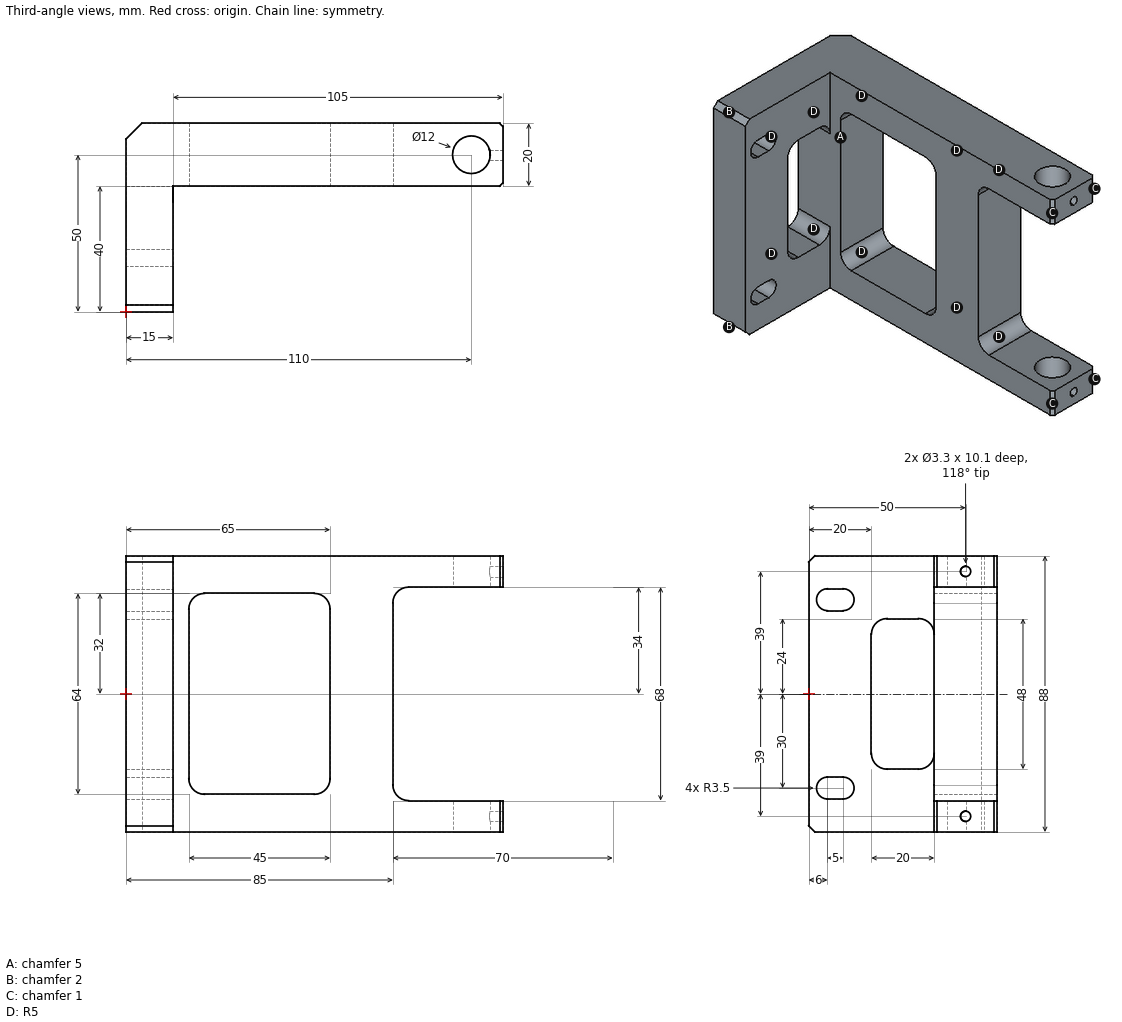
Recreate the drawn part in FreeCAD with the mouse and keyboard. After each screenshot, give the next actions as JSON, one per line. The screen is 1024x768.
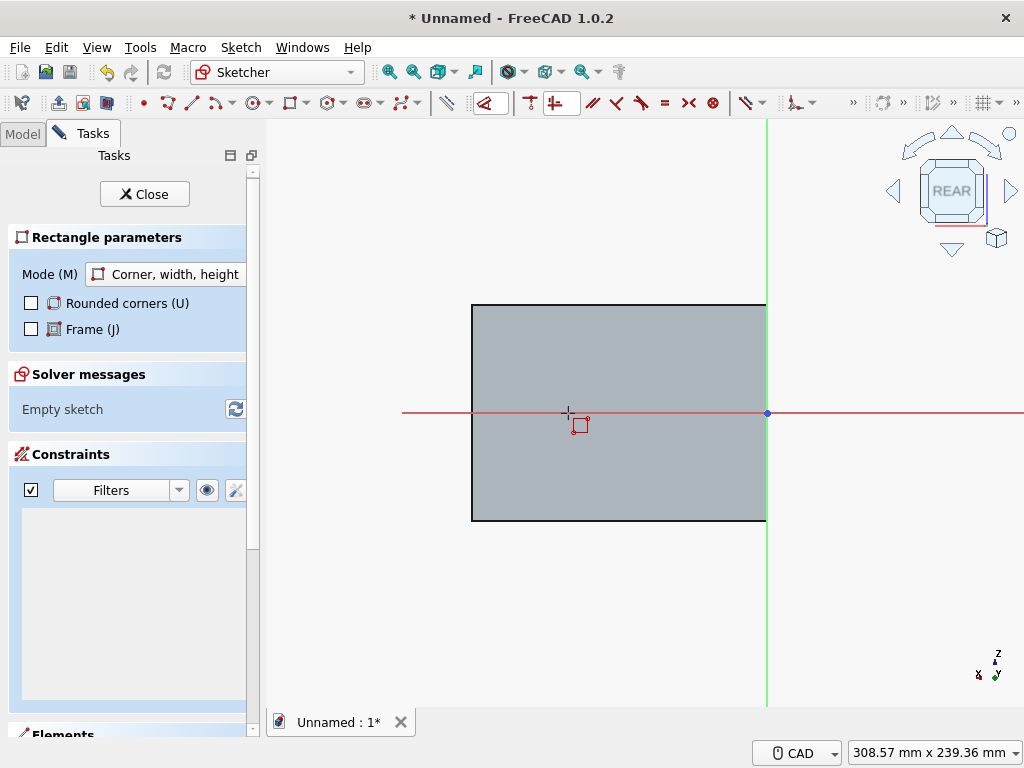
{"action": "left_click", "coordinate": [386, 330]}
{"action": "mouse_move", "coordinate": [558, 497]}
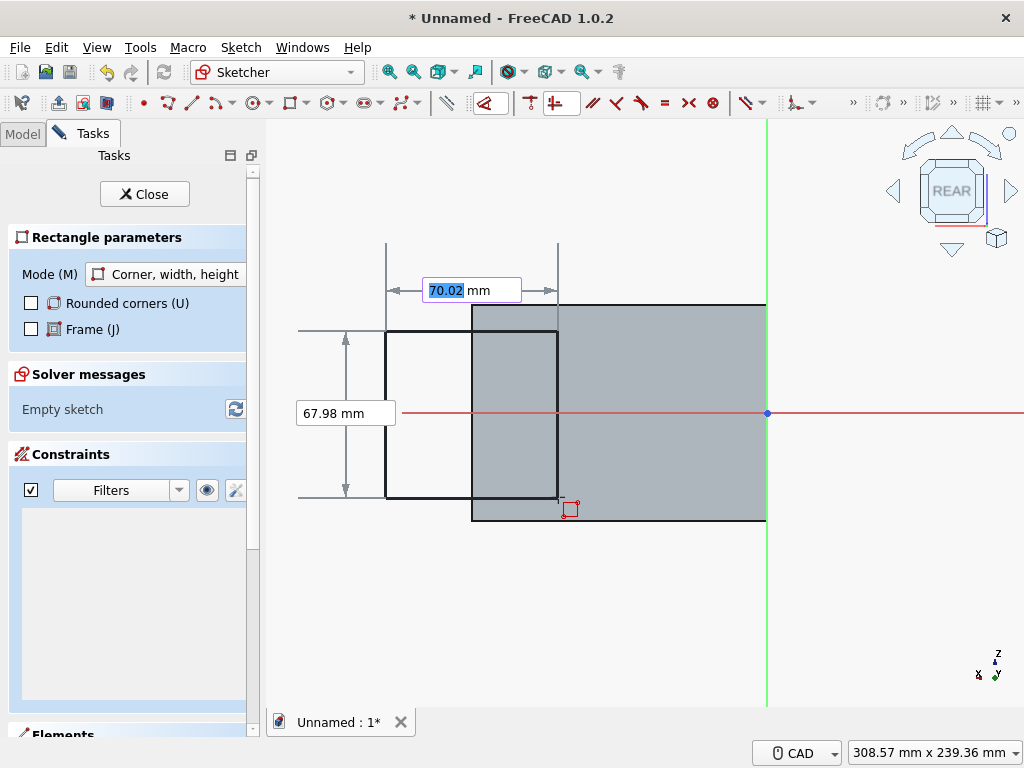
{"action": "type", "text": "70"}
{"action": "key", "text": "Tab"}
{"action": "type", "text": "68"}
{"action": "key", "text": "Return"}
{"action": "key", "text": "Escape"}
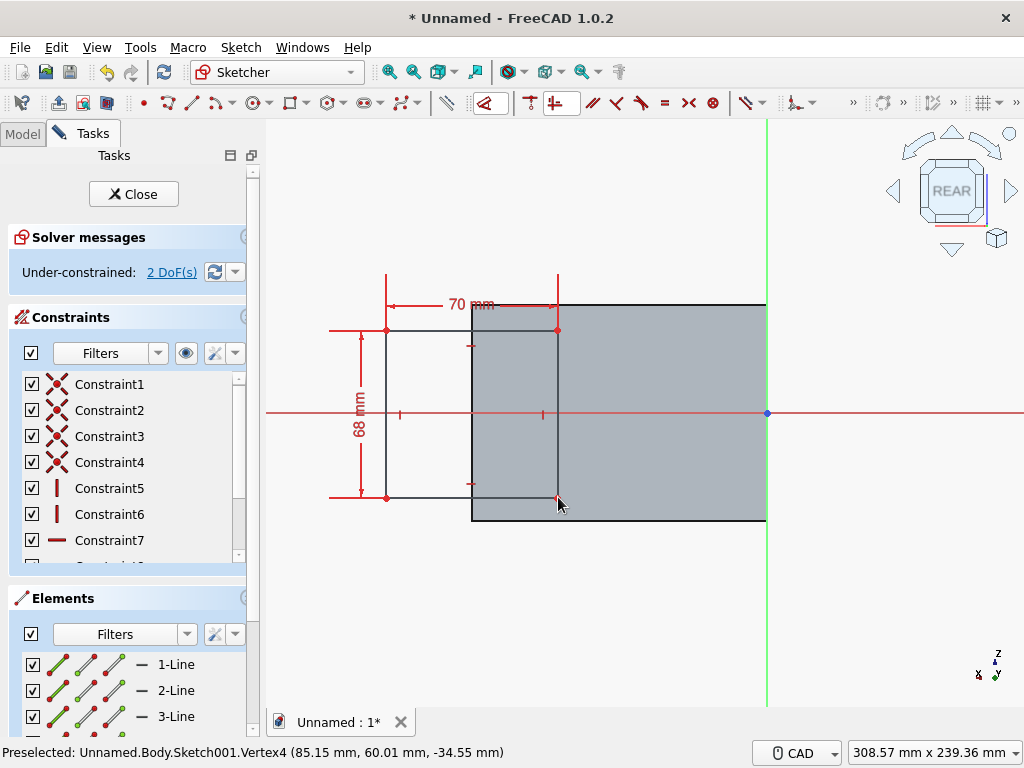
{"action": "left_click", "coordinate": [386, 331]}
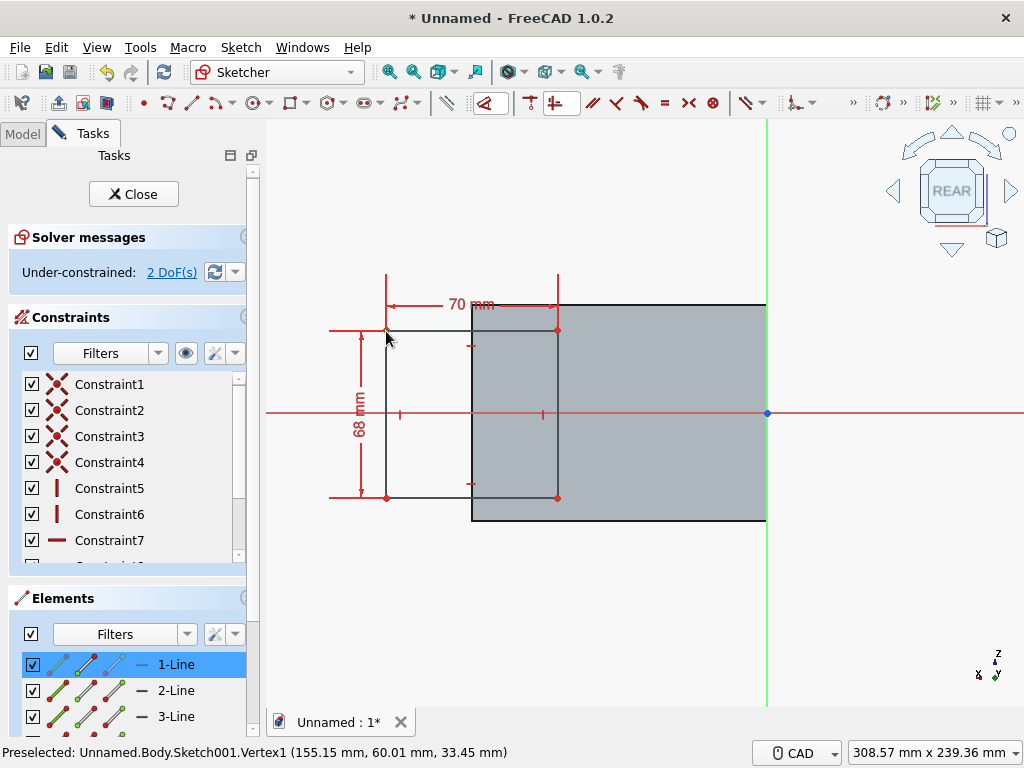
{"action": "key", "text": "i"}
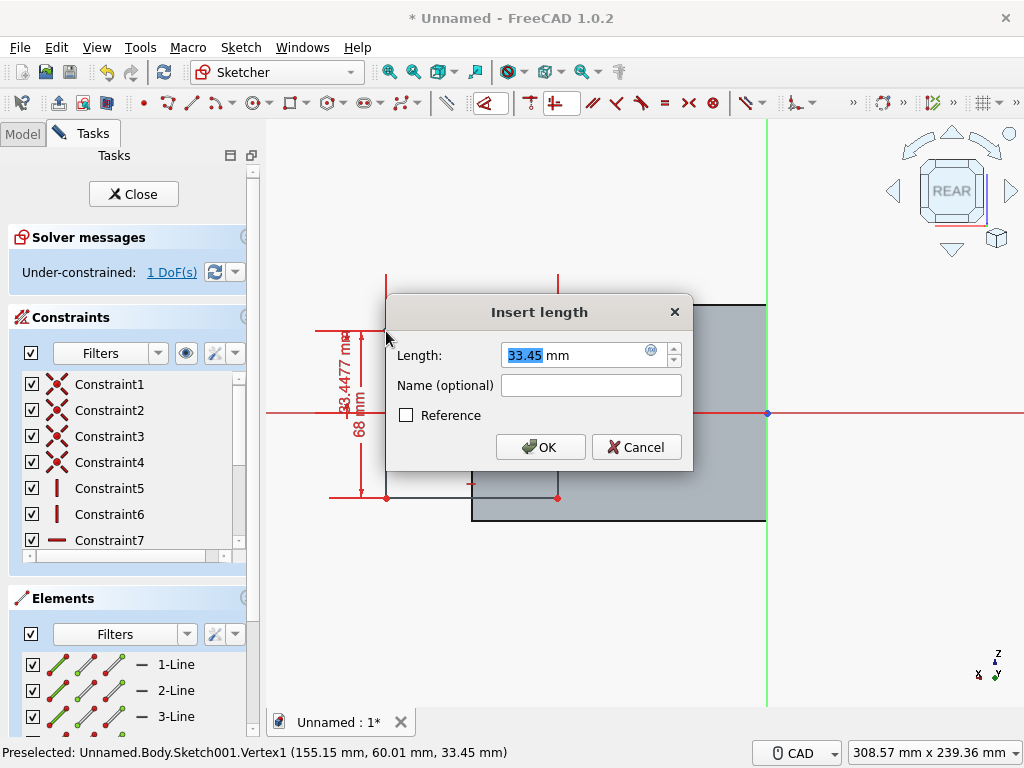
{"action": "type", "text": "34"}
{"action": "key", "text": "Return"}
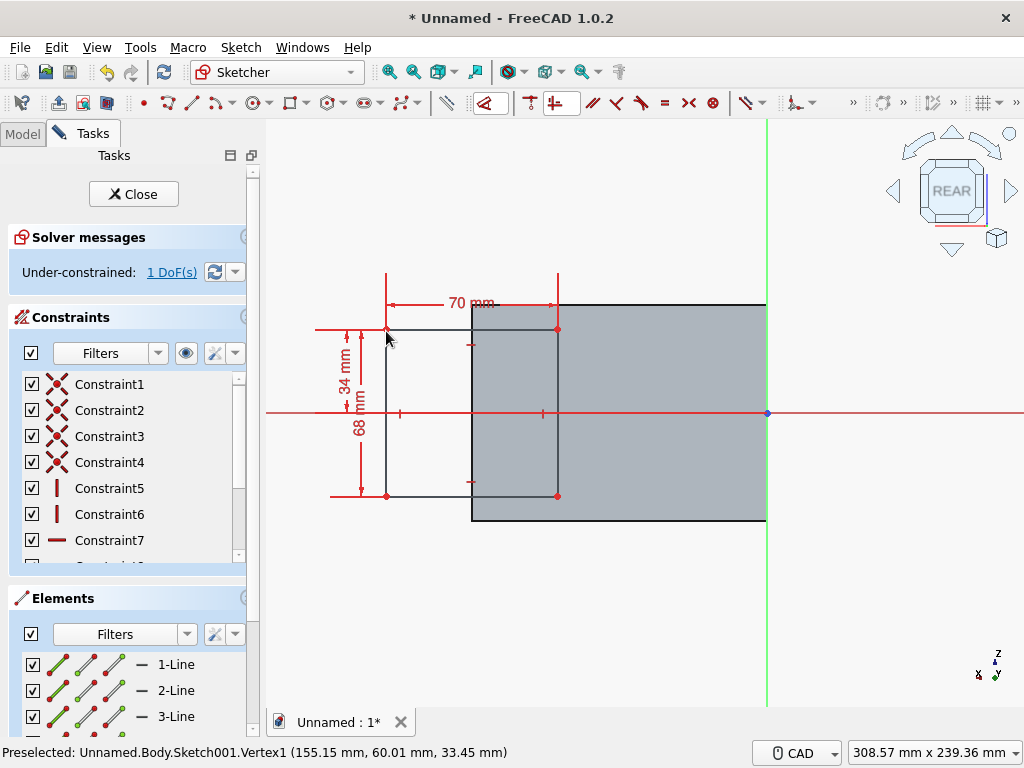
{"action": "left_click", "coordinate": [558, 497]}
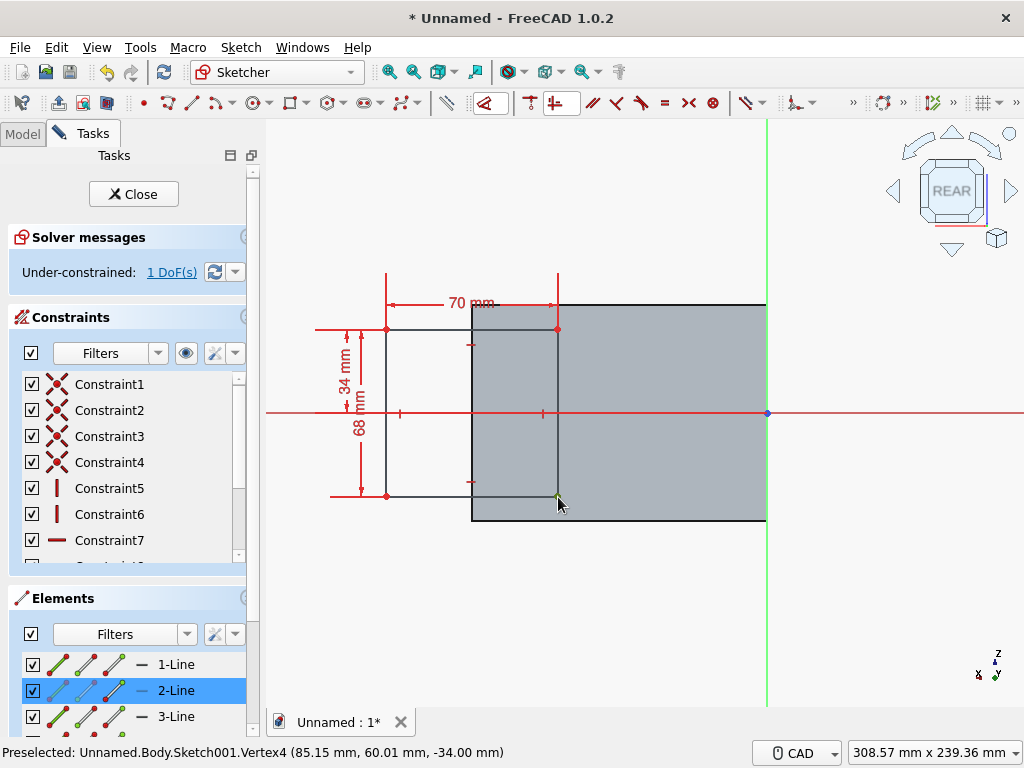
{"action": "key", "text": "l"}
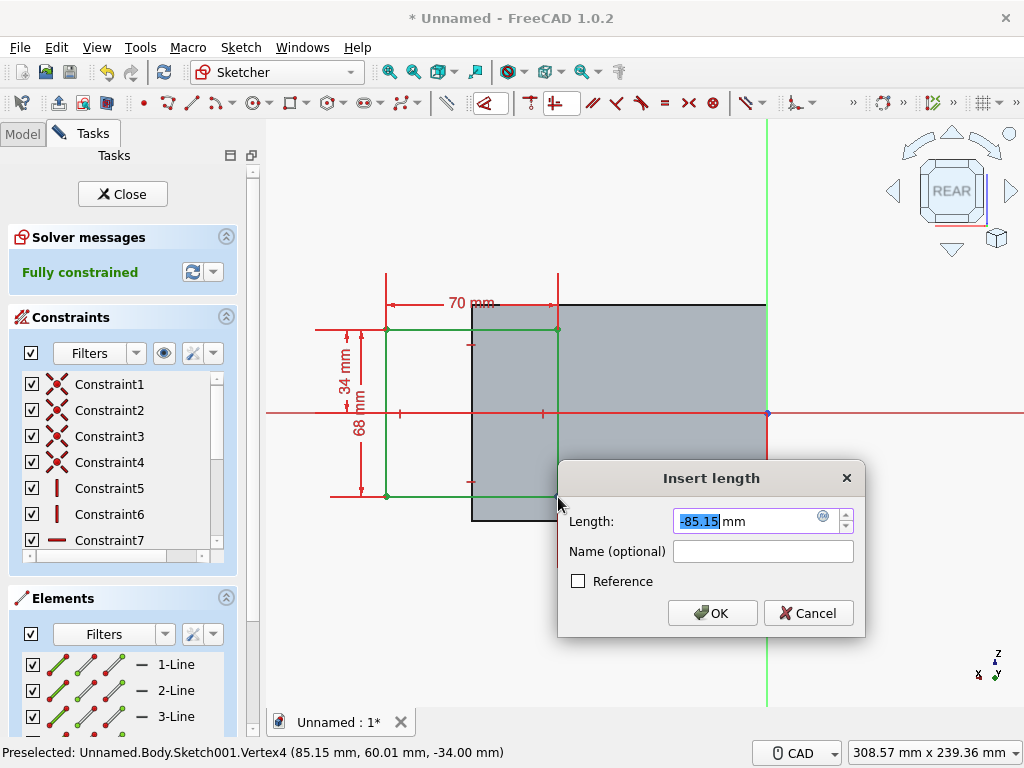
{"action": "type", "text": "-85"}
{"action": "key", "text": "Return"}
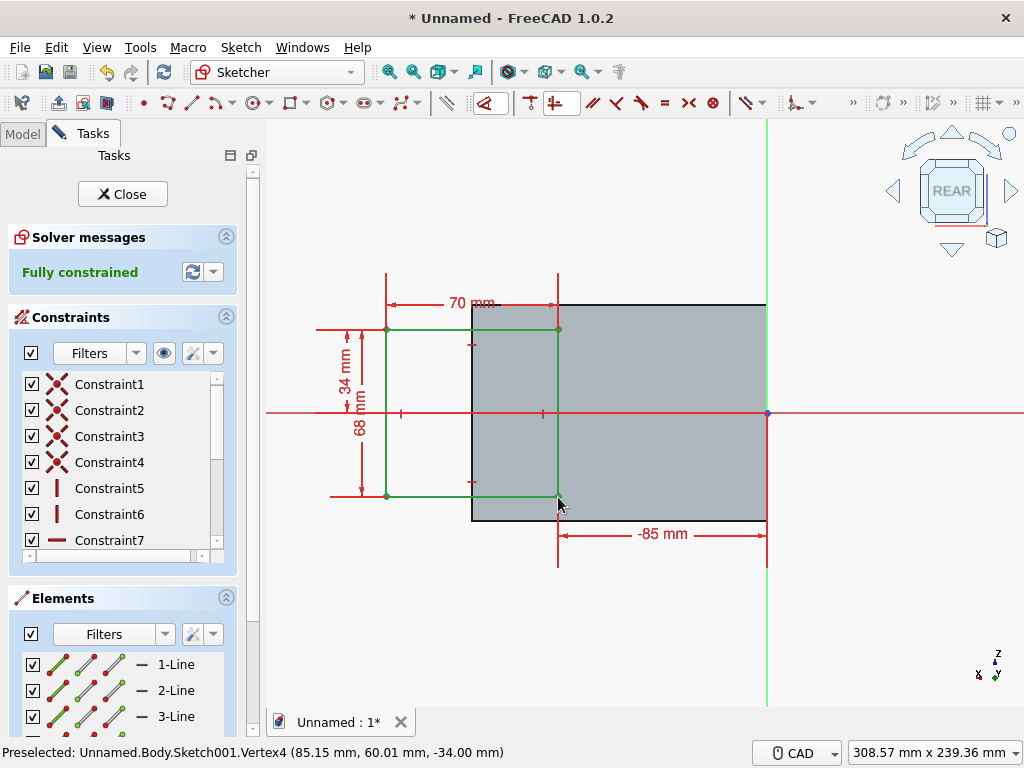
{"action": "left_click", "coordinate": [123, 194]}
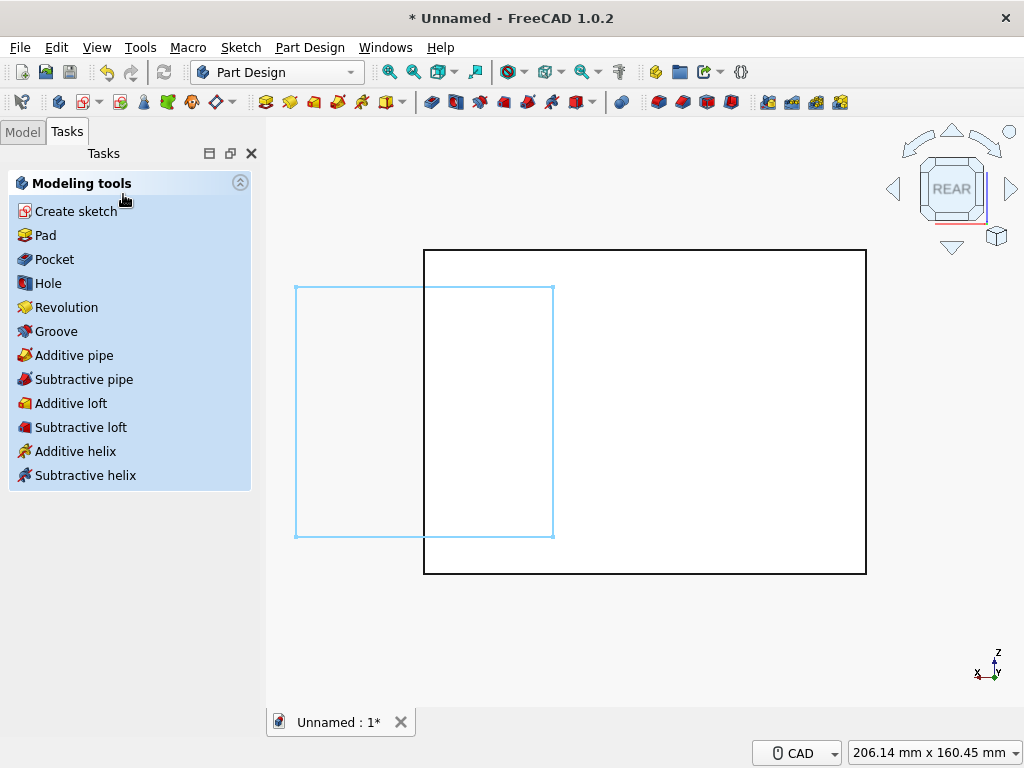
{"action": "left_click", "coordinate": [432, 102]}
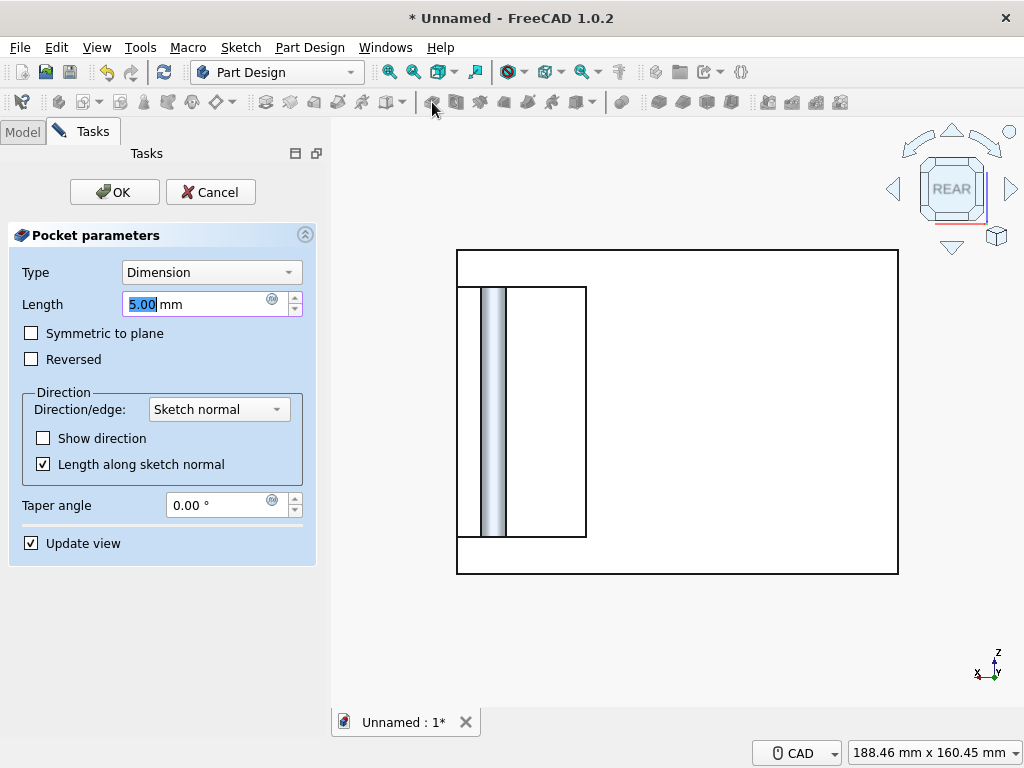
{"action": "left_click", "coordinate": [212, 272]}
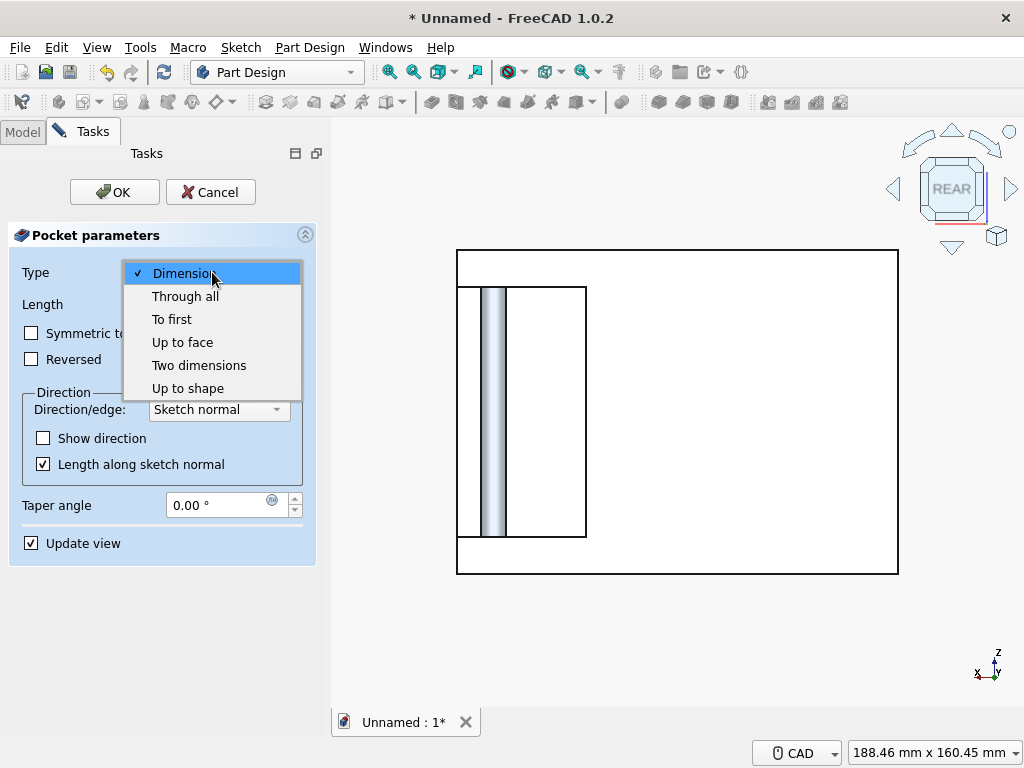
{"action": "left_click", "coordinate": [212, 296]}